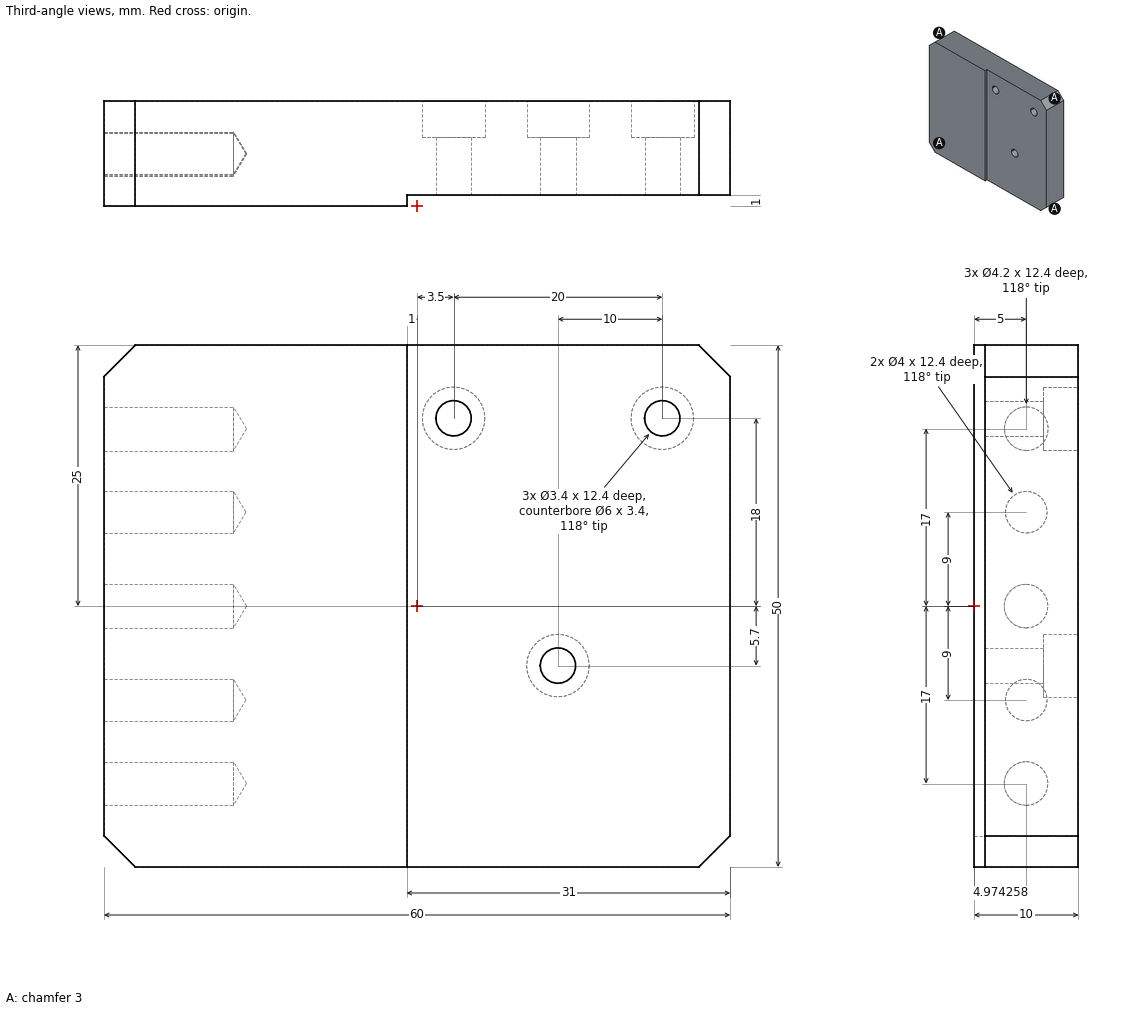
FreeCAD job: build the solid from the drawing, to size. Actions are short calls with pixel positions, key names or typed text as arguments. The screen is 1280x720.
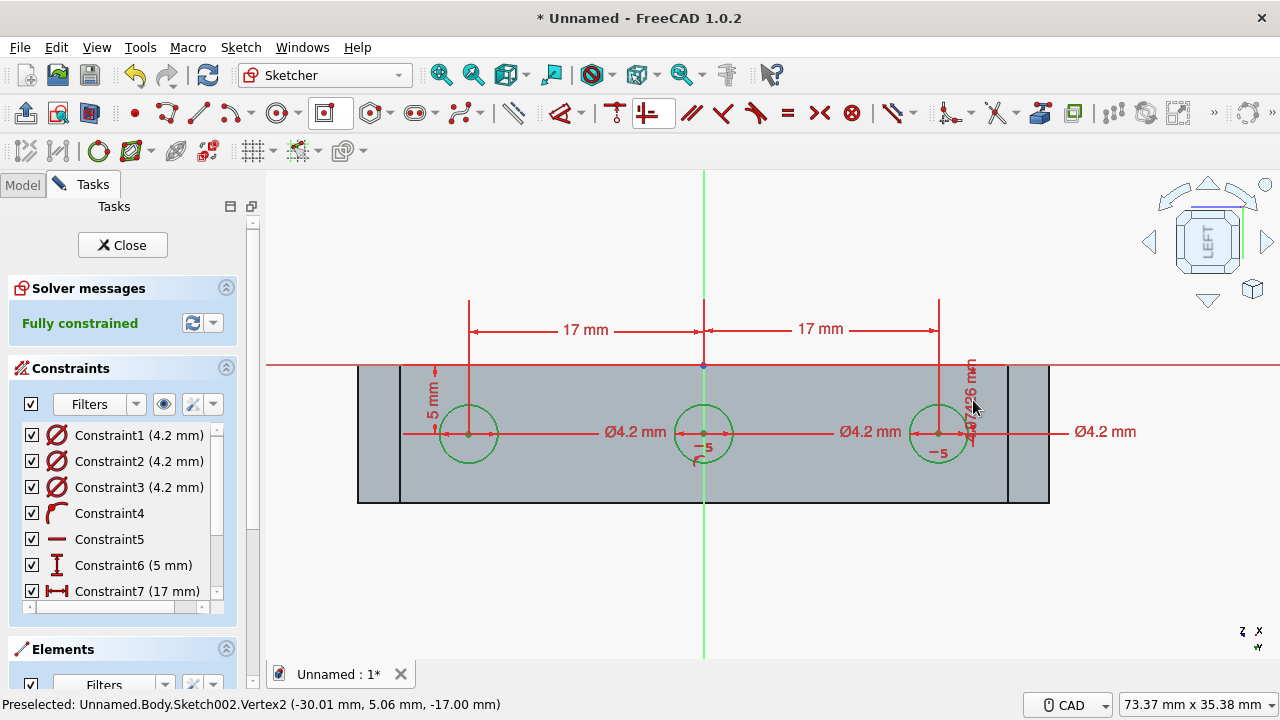
click(123, 245)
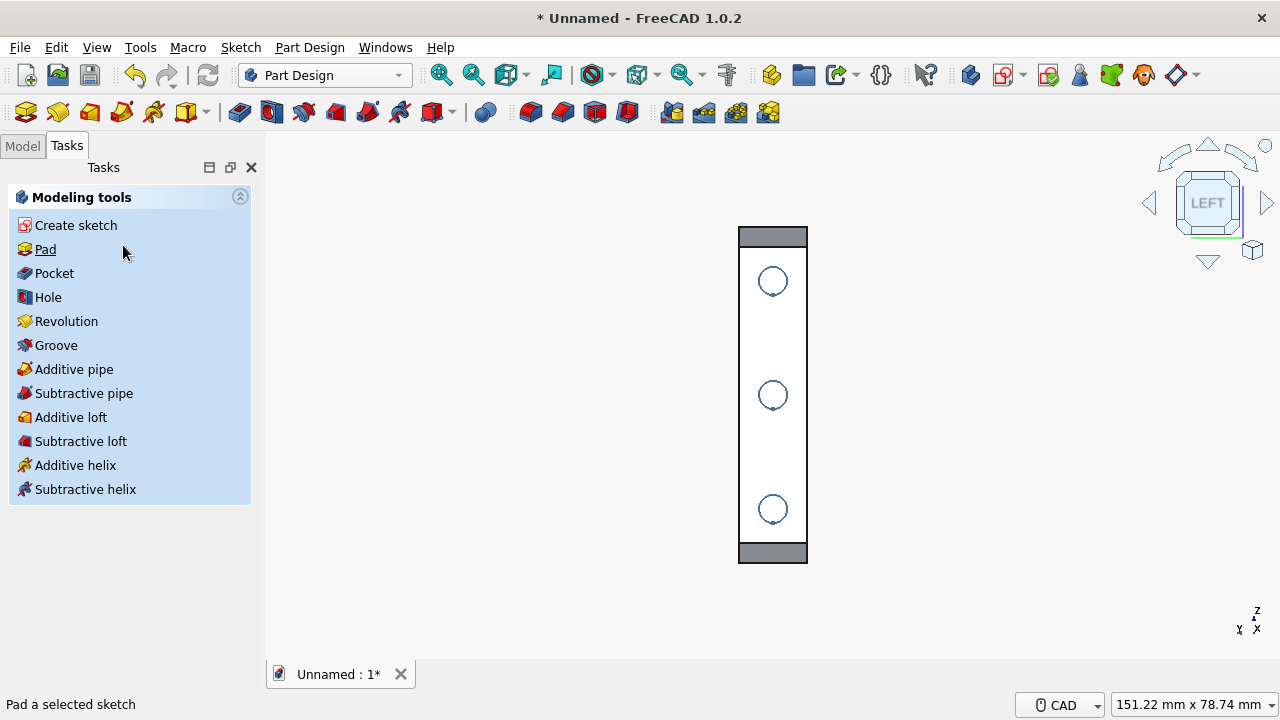
click(272, 112)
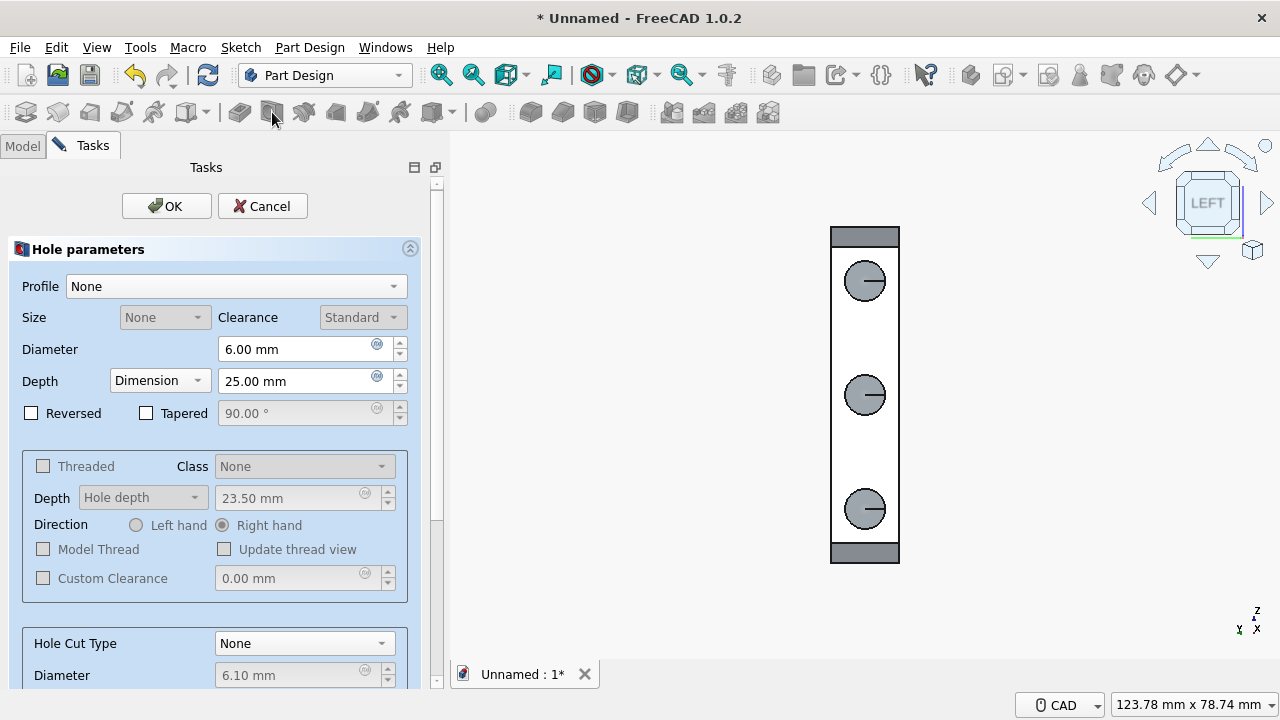
triple_click(305, 349)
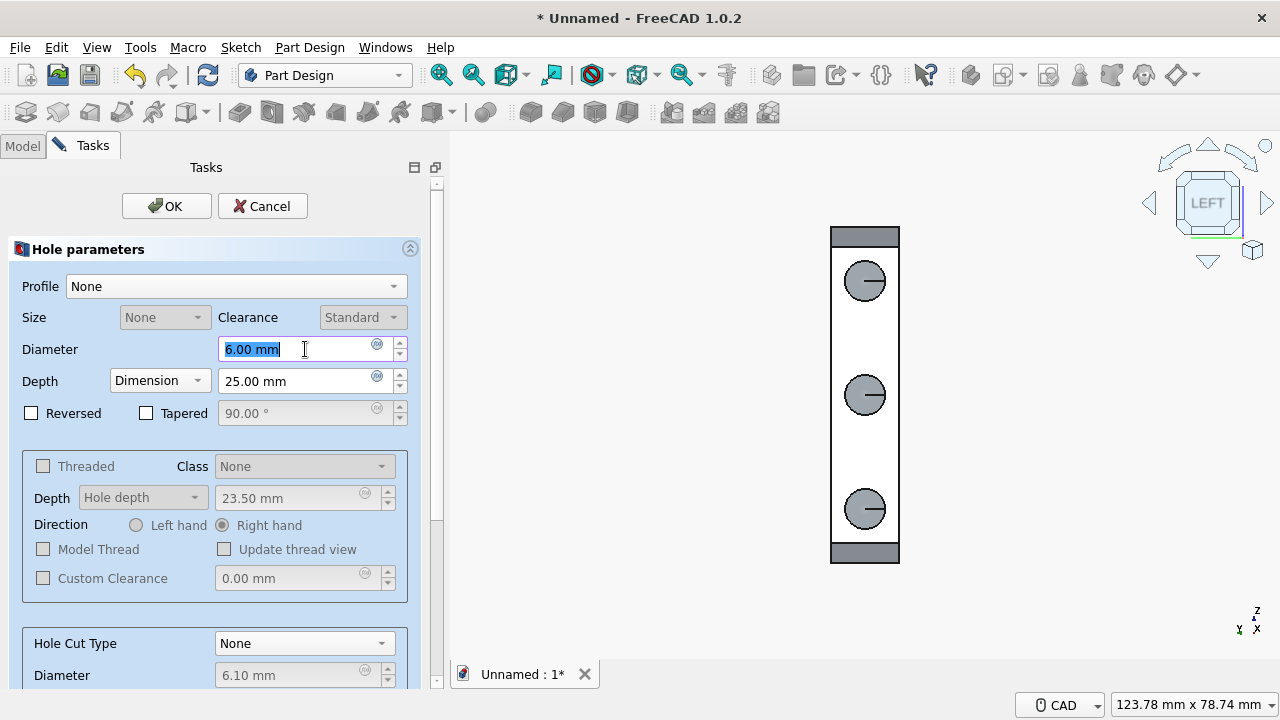
text(4.2)
key(Tab)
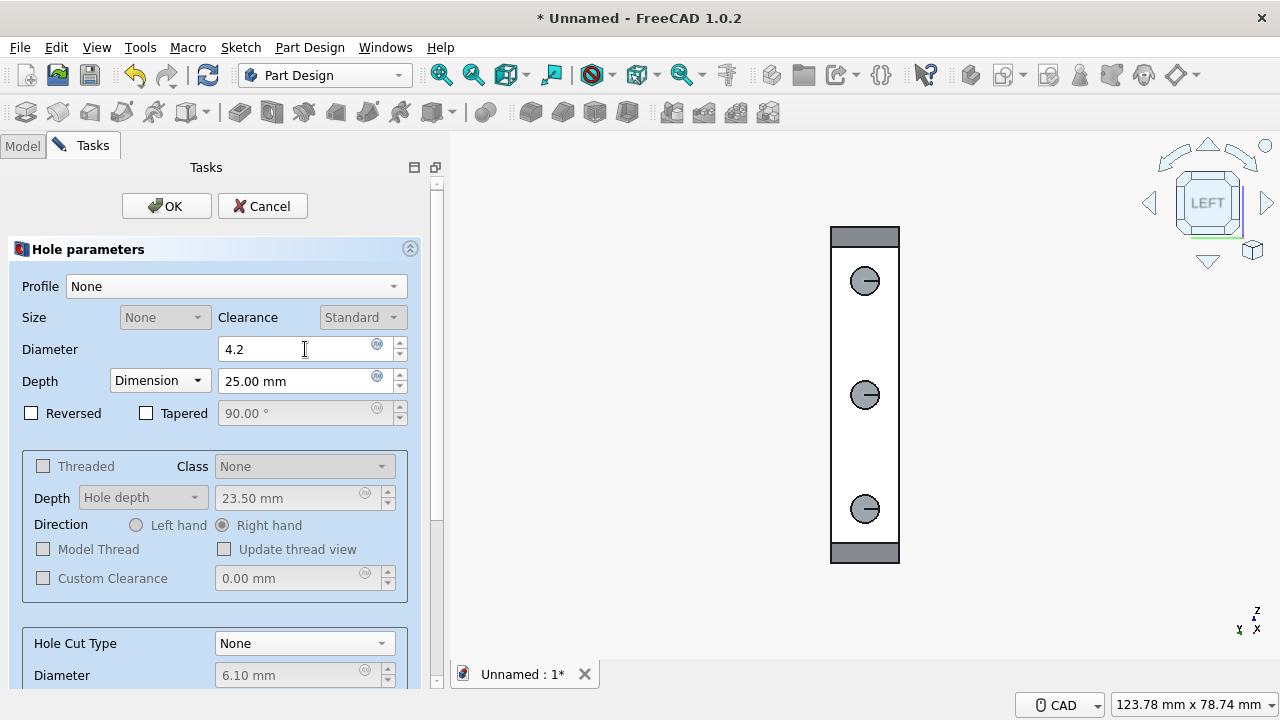
triple_click(305, 381)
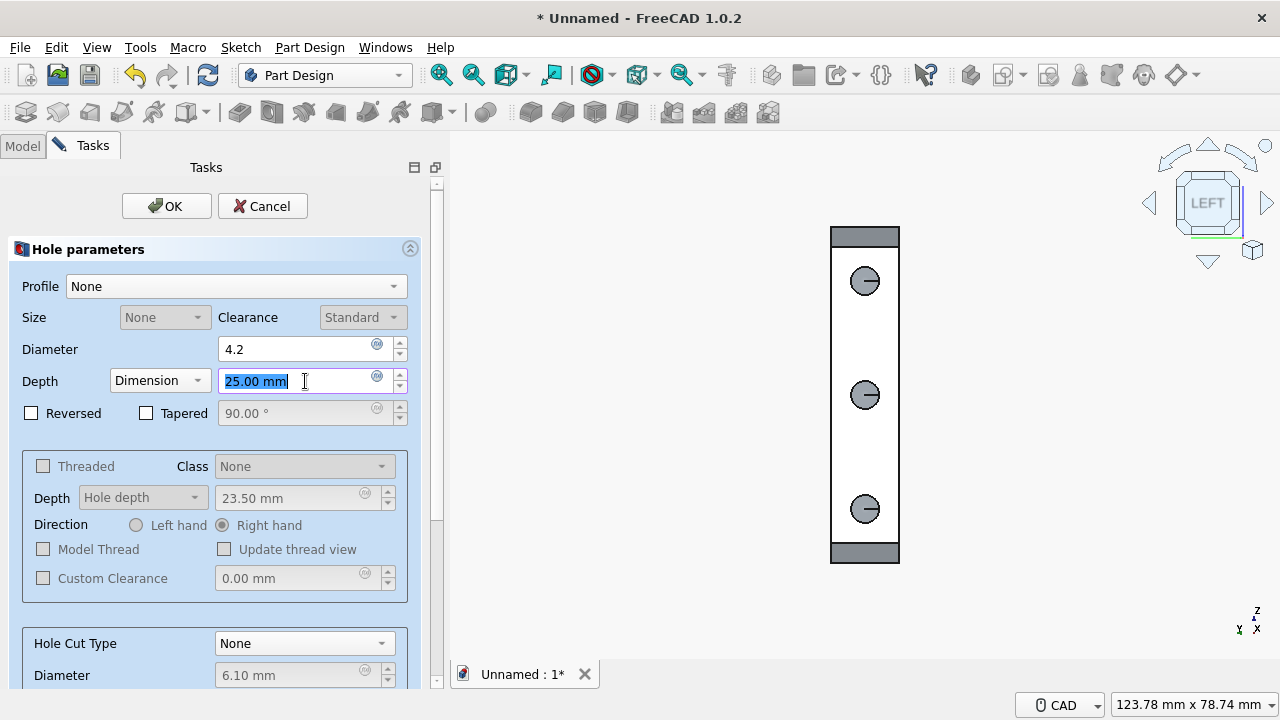
text(12.4)
key(Tab)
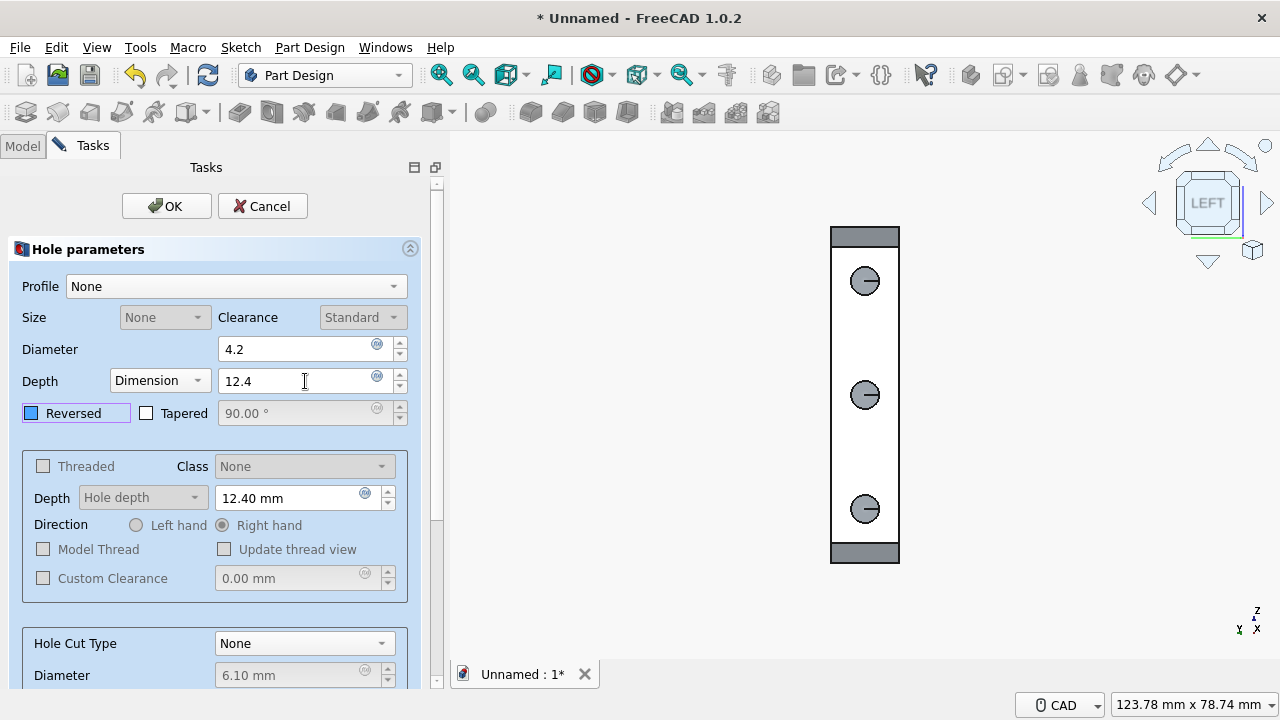
click(167, 206)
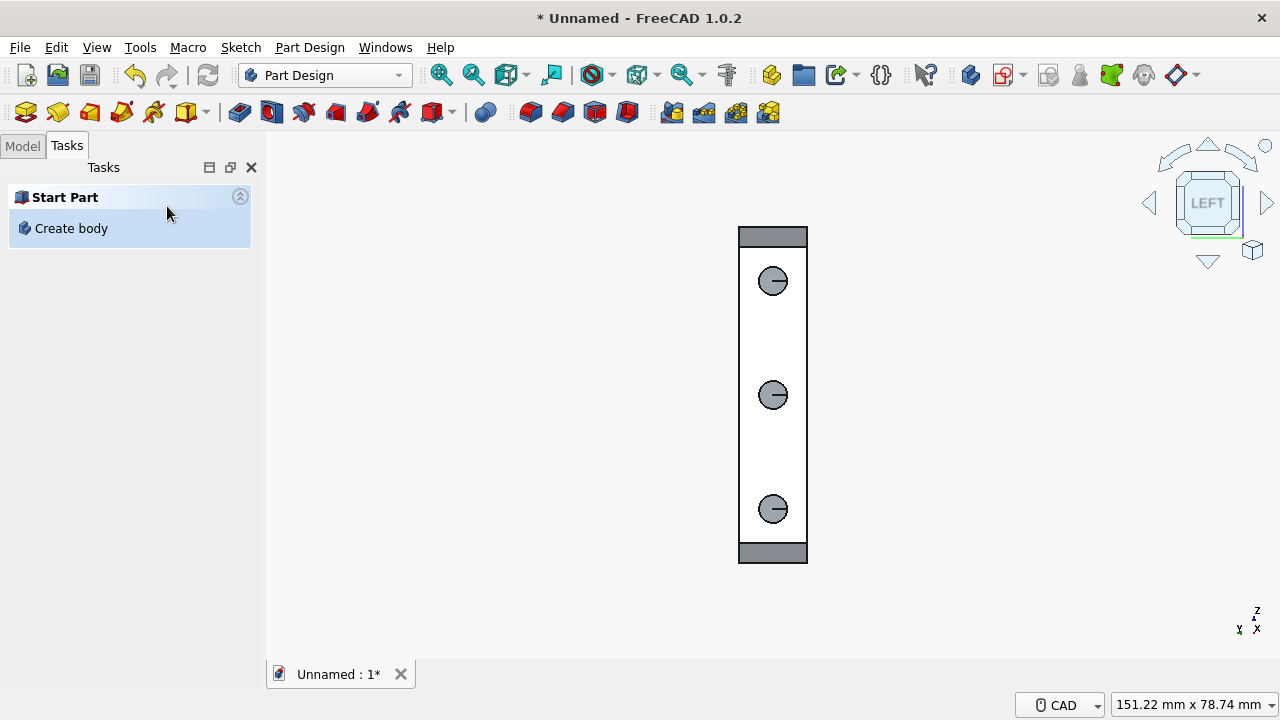
key(4)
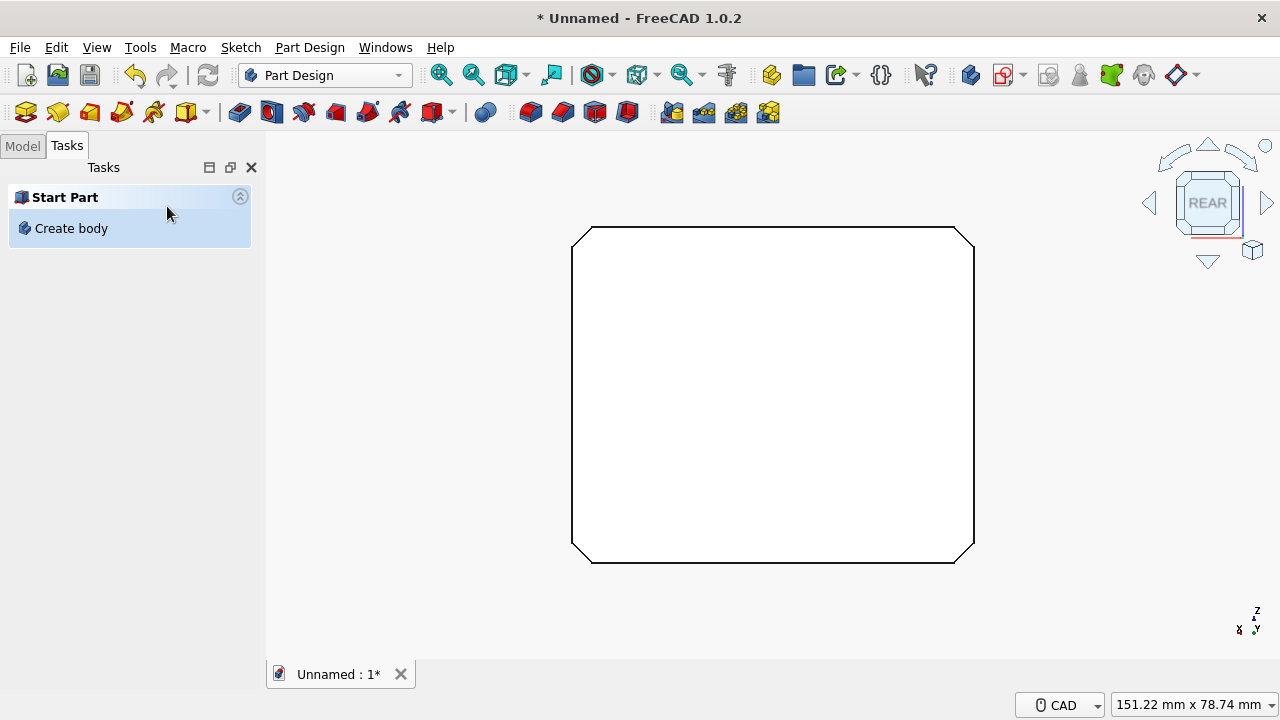
click(773, 394)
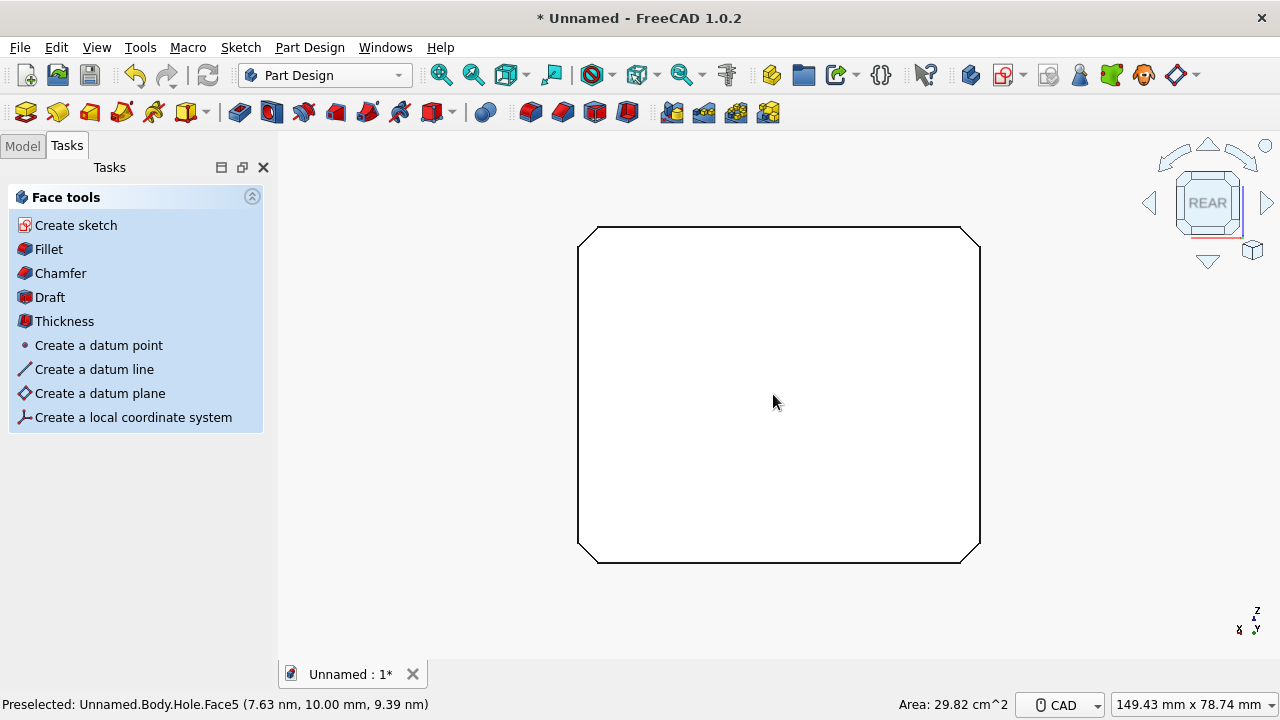
click(1004, 76)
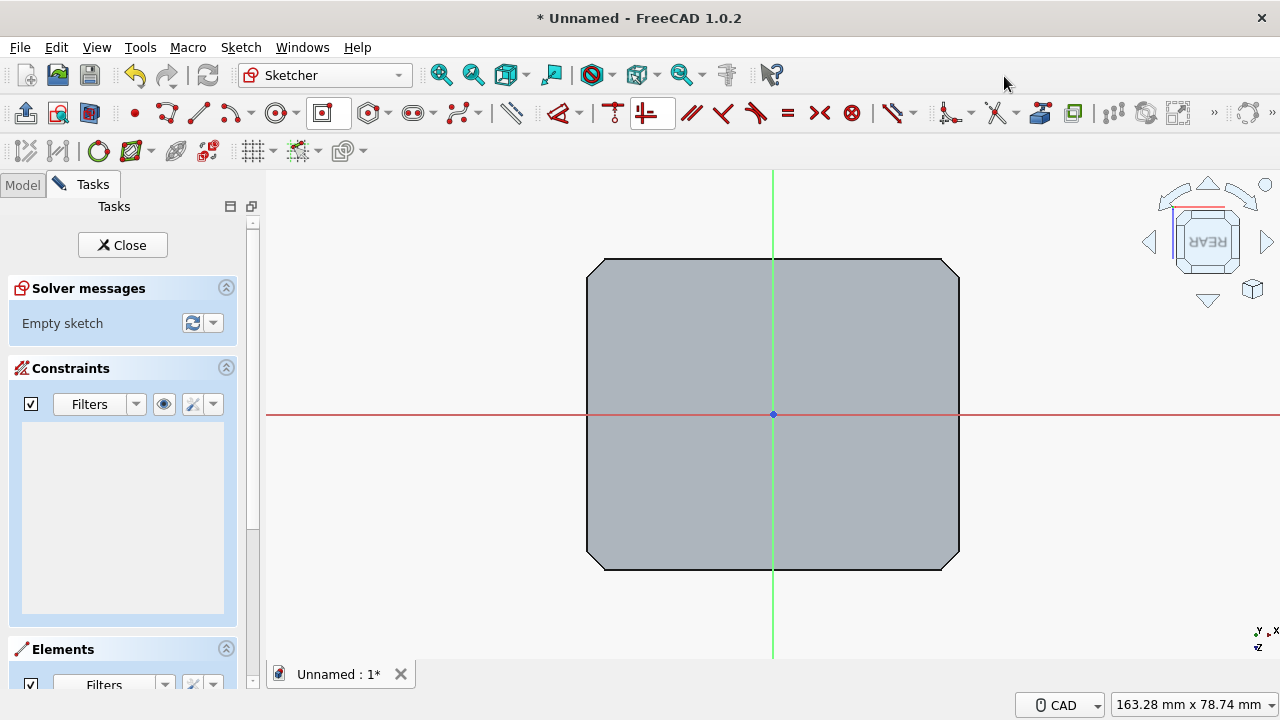
scroll(1030, 499, up, 3)